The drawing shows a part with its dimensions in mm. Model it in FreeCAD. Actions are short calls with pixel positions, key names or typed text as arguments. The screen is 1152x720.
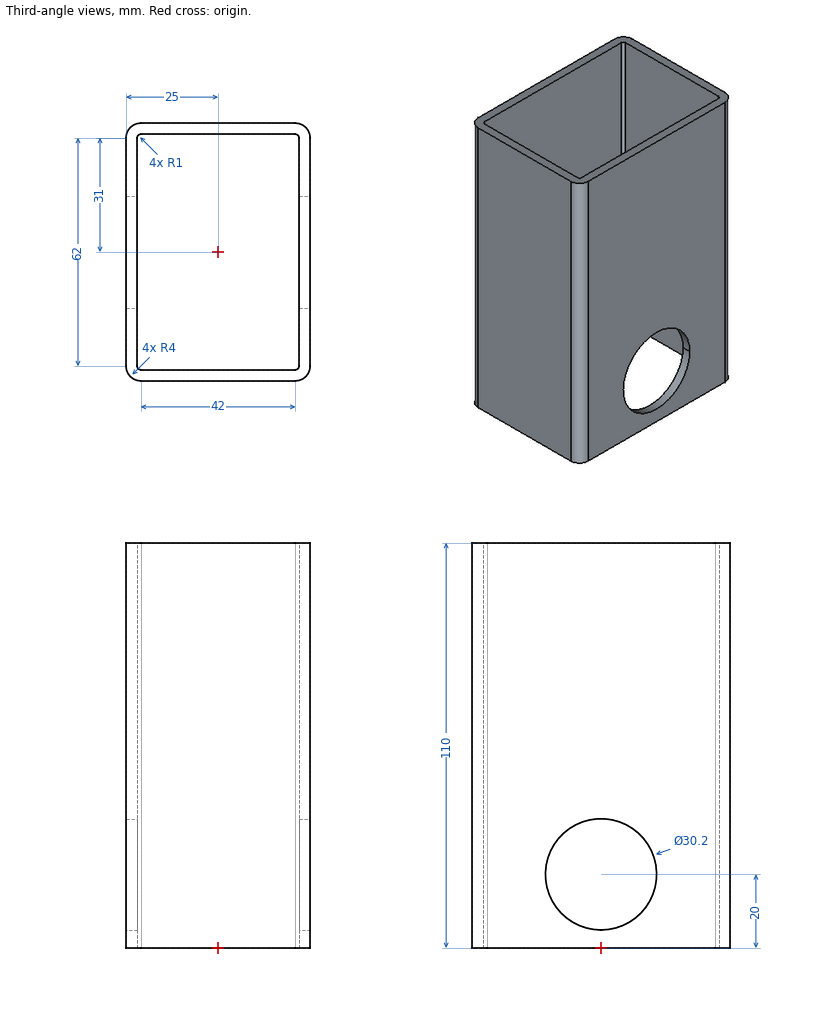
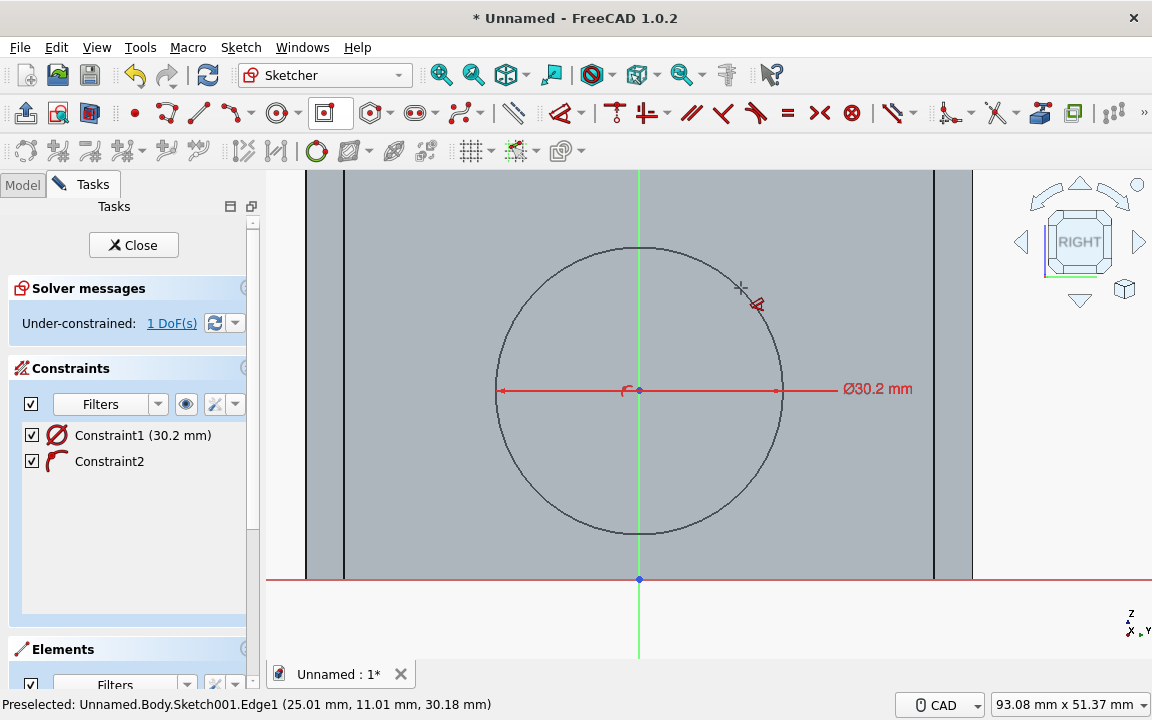
click(639, 391)
click(673, 485)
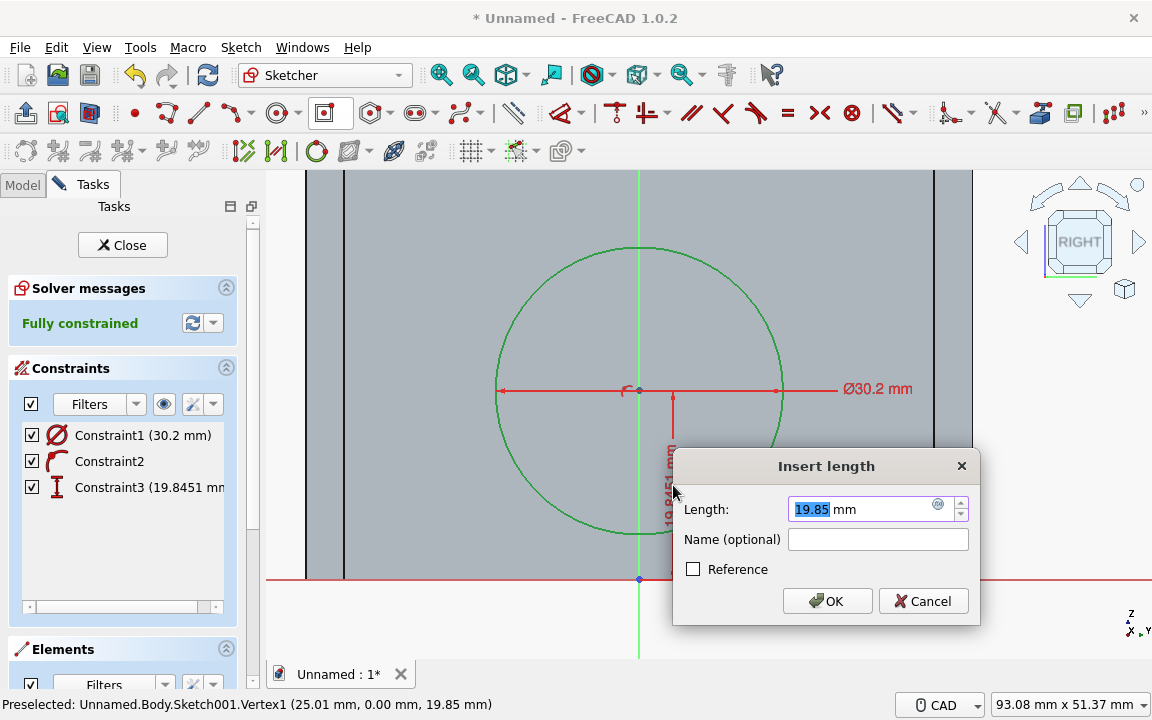
text(20)
key(Return)
key(Escape)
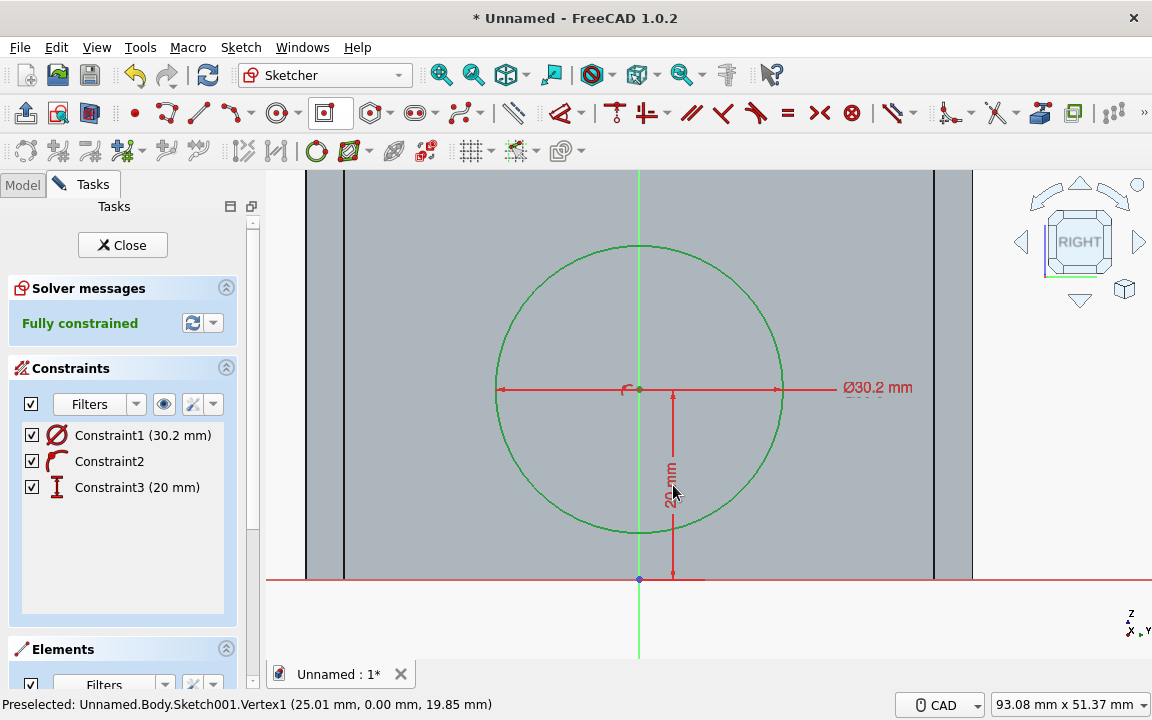
click(123, 245)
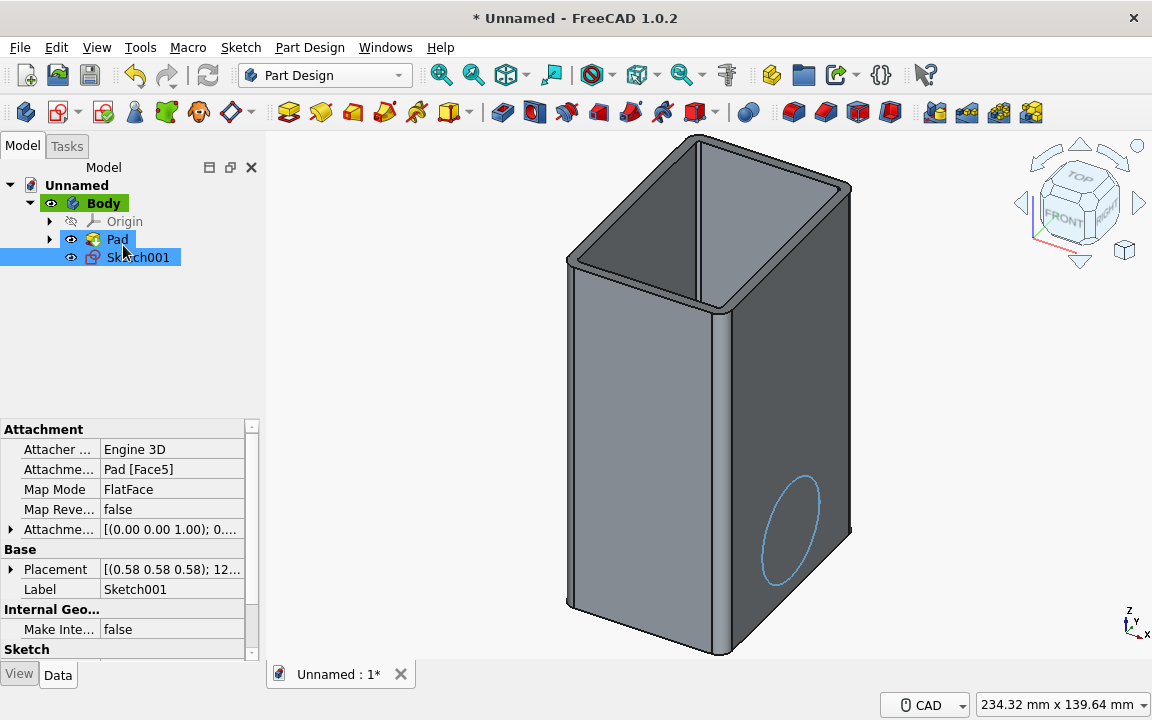
click(504, 112)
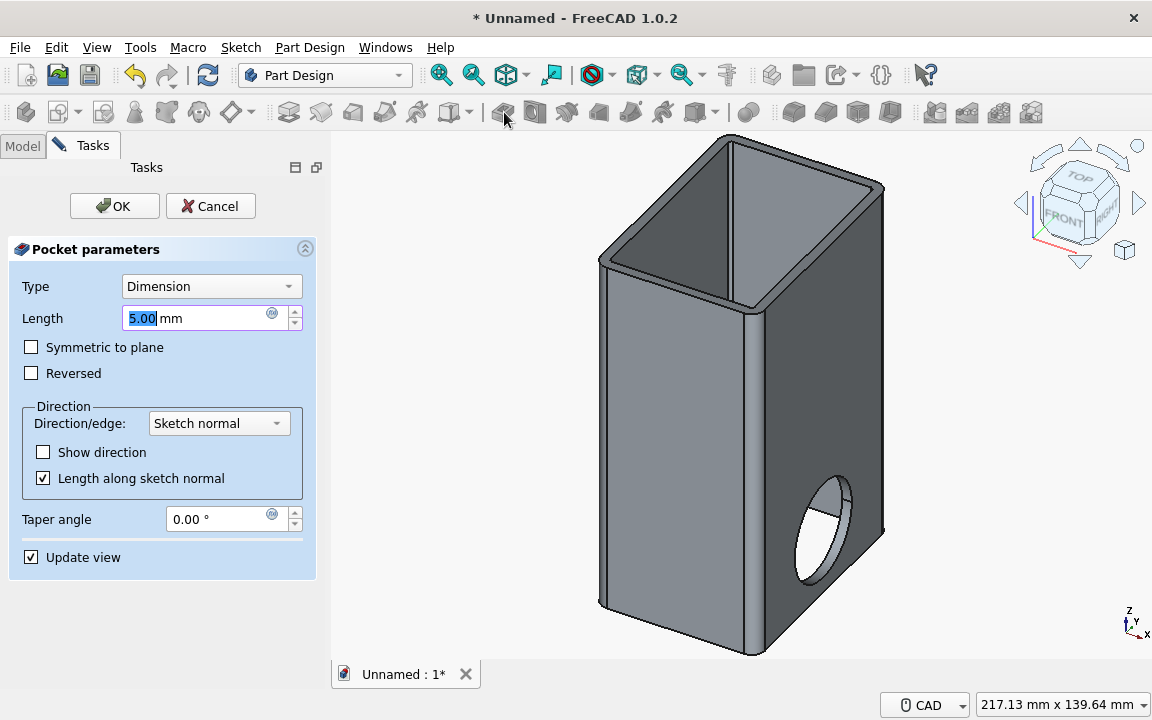
click(212, 286)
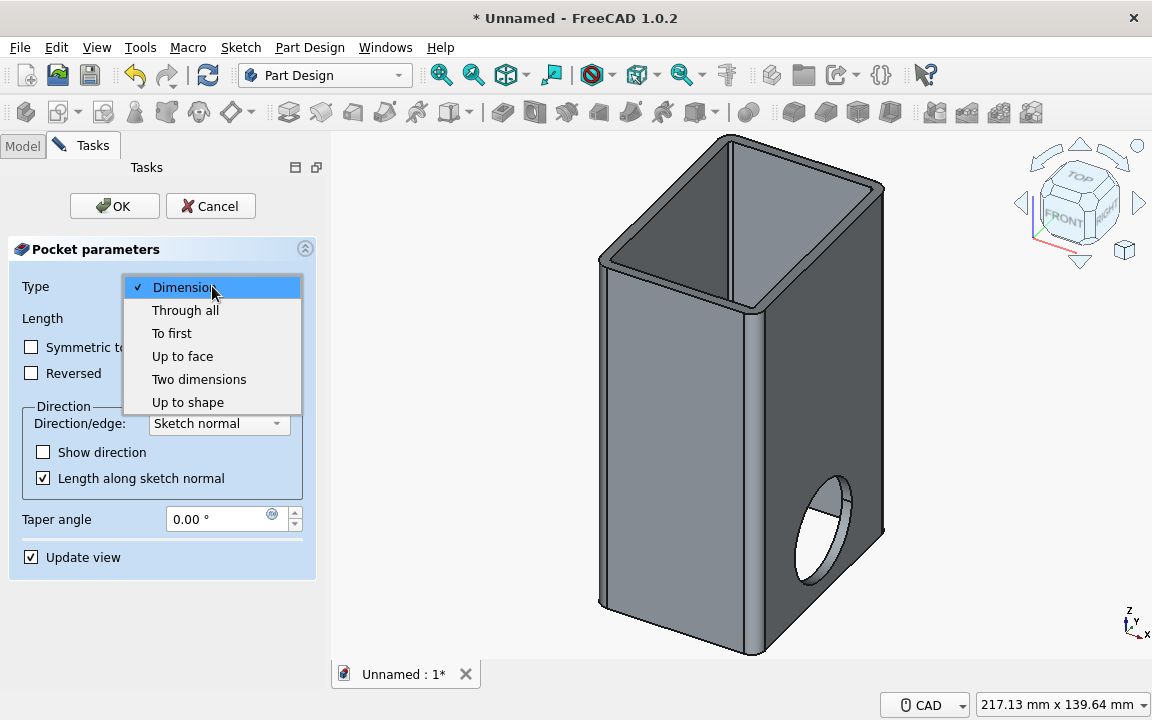
click(212, 310)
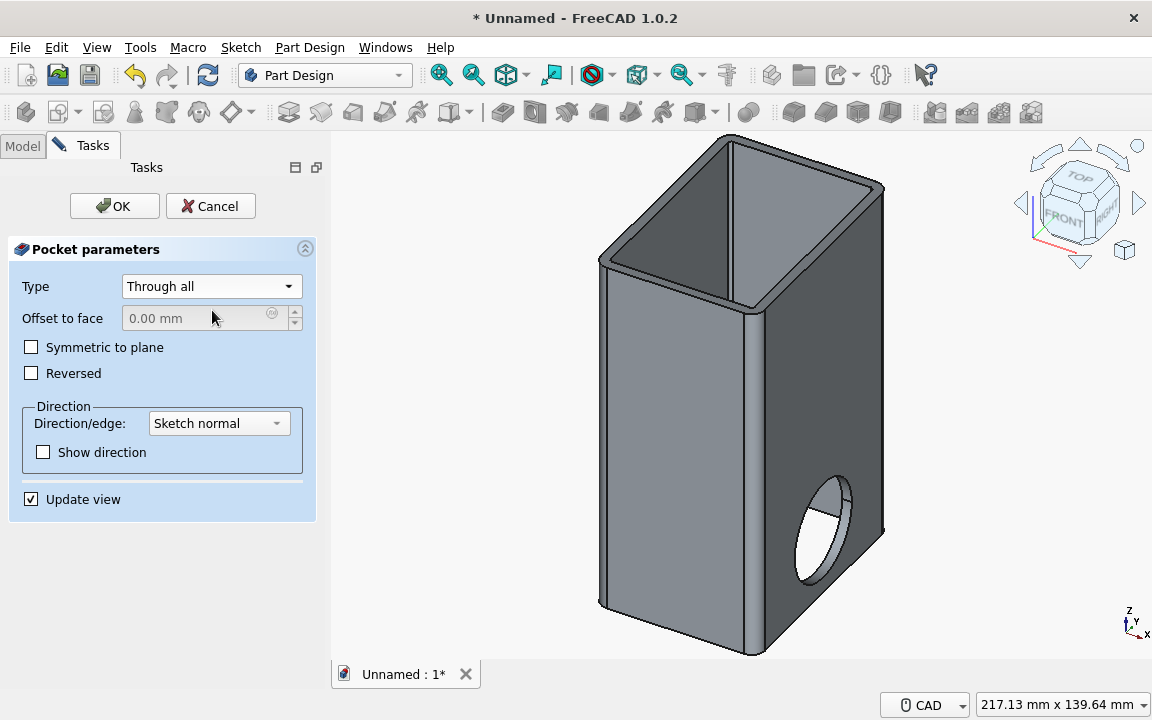
click(115, 206)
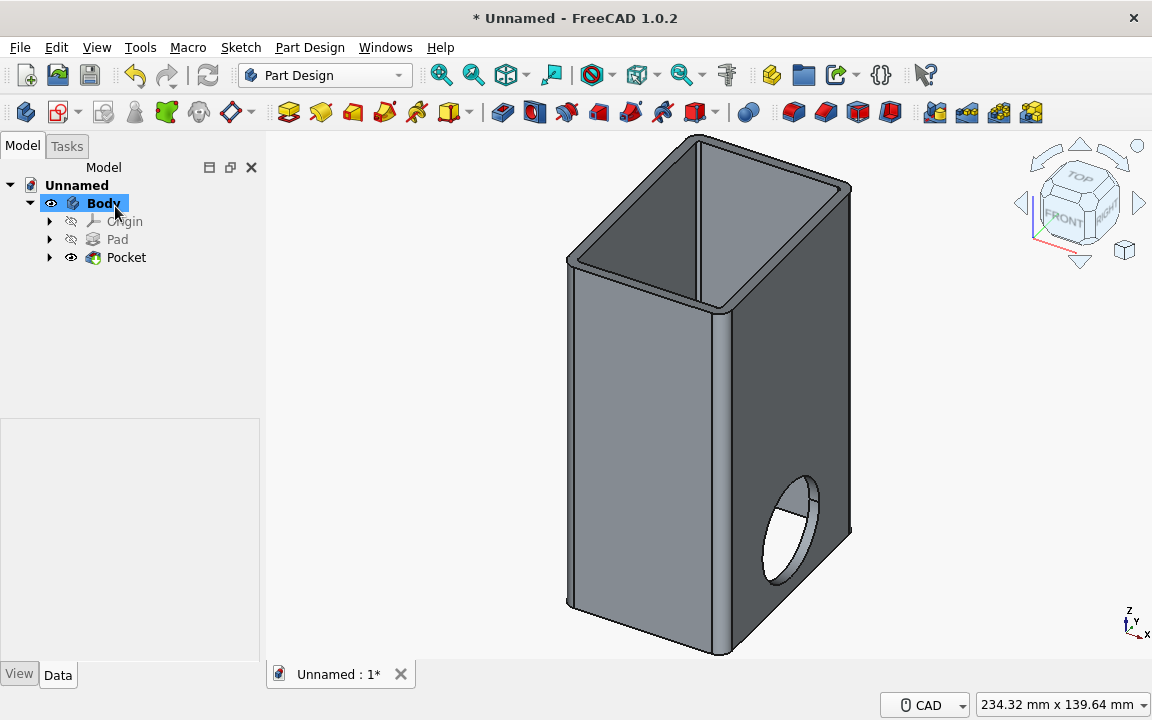
key(0)